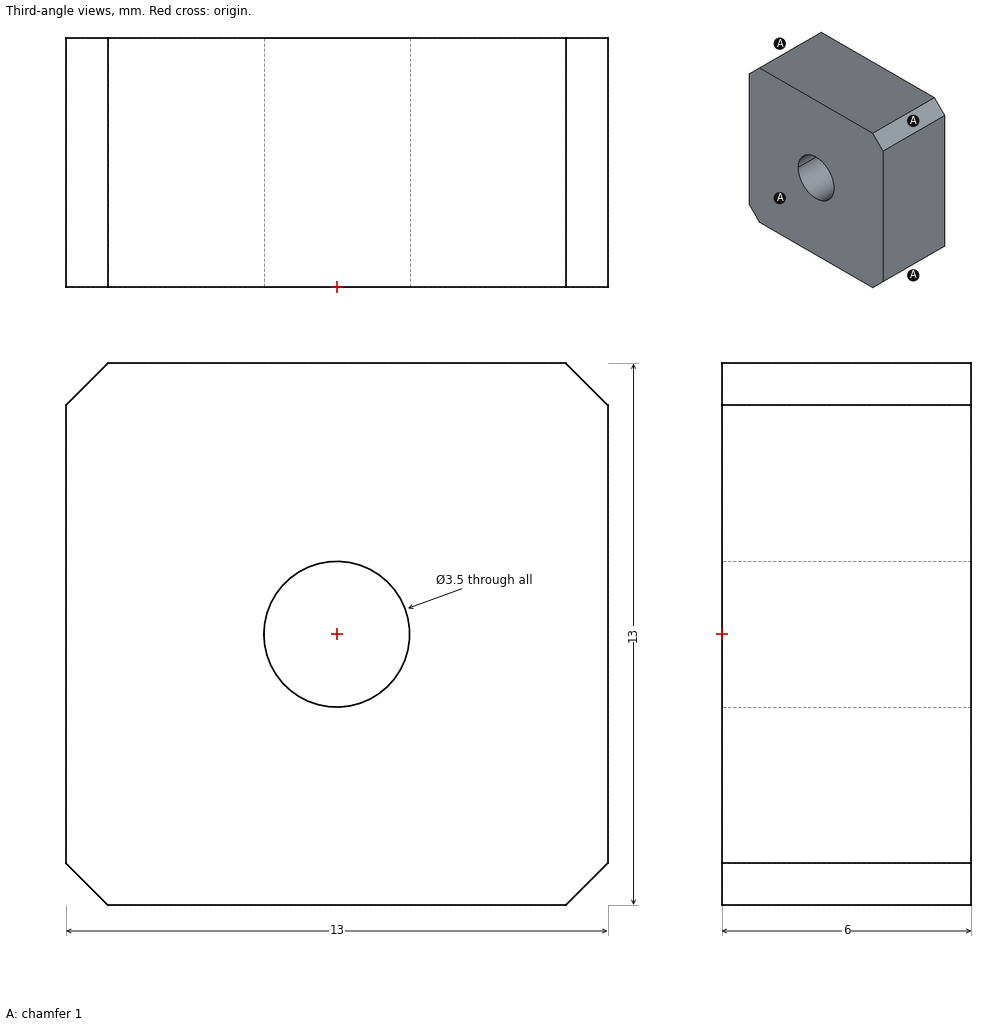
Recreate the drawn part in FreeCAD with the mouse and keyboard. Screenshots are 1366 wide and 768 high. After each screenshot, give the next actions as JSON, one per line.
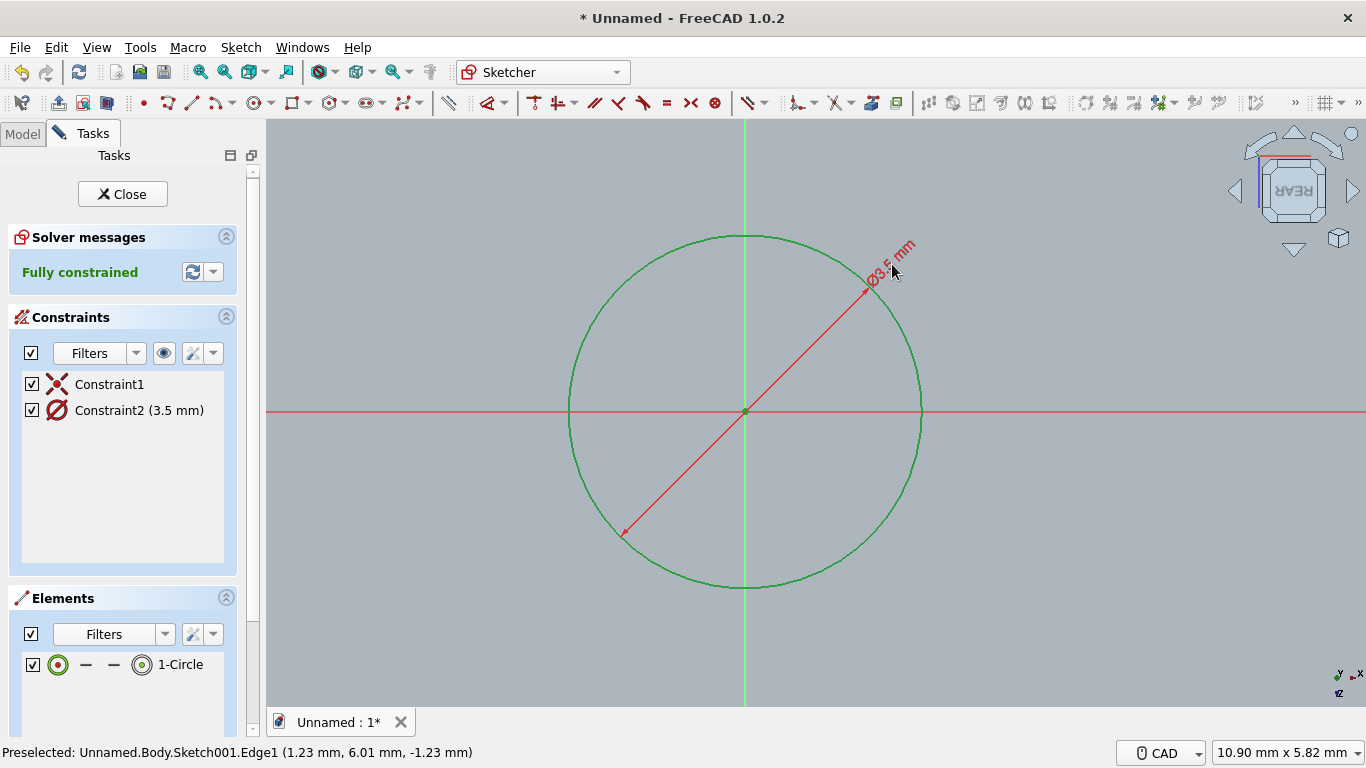
{"action": "left_click", "coordinate": [123, 194]}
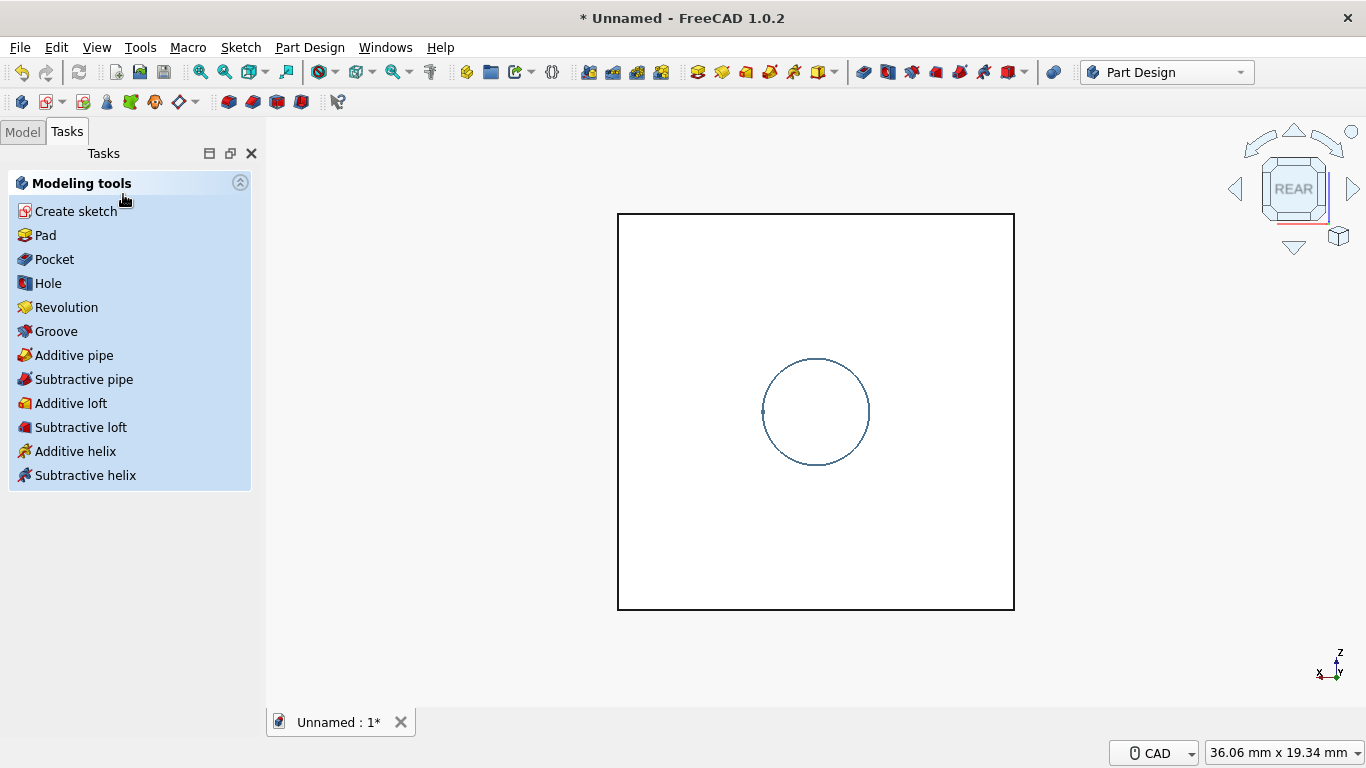
{"action": "left_click", "coordinate": [888, 72]}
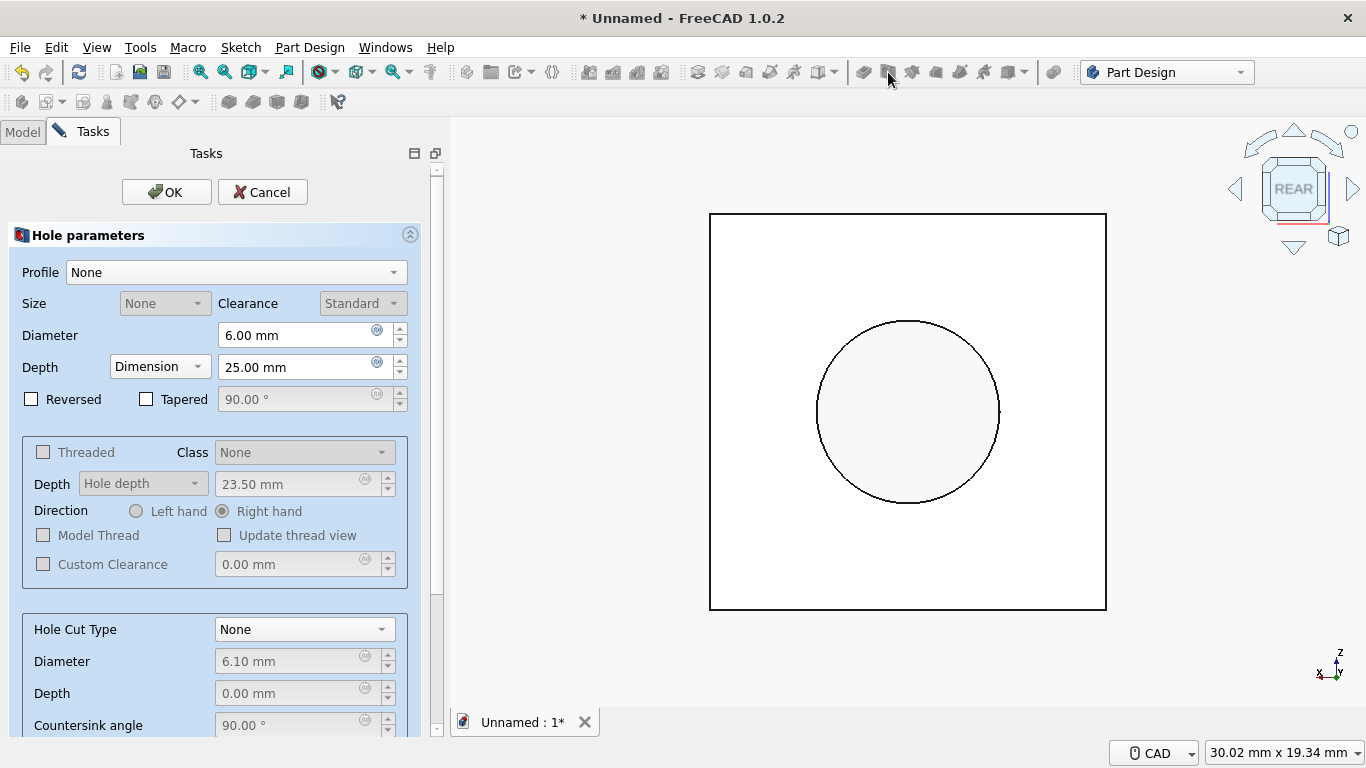
{"action": "triple_click", "coordinate": [305, 335]}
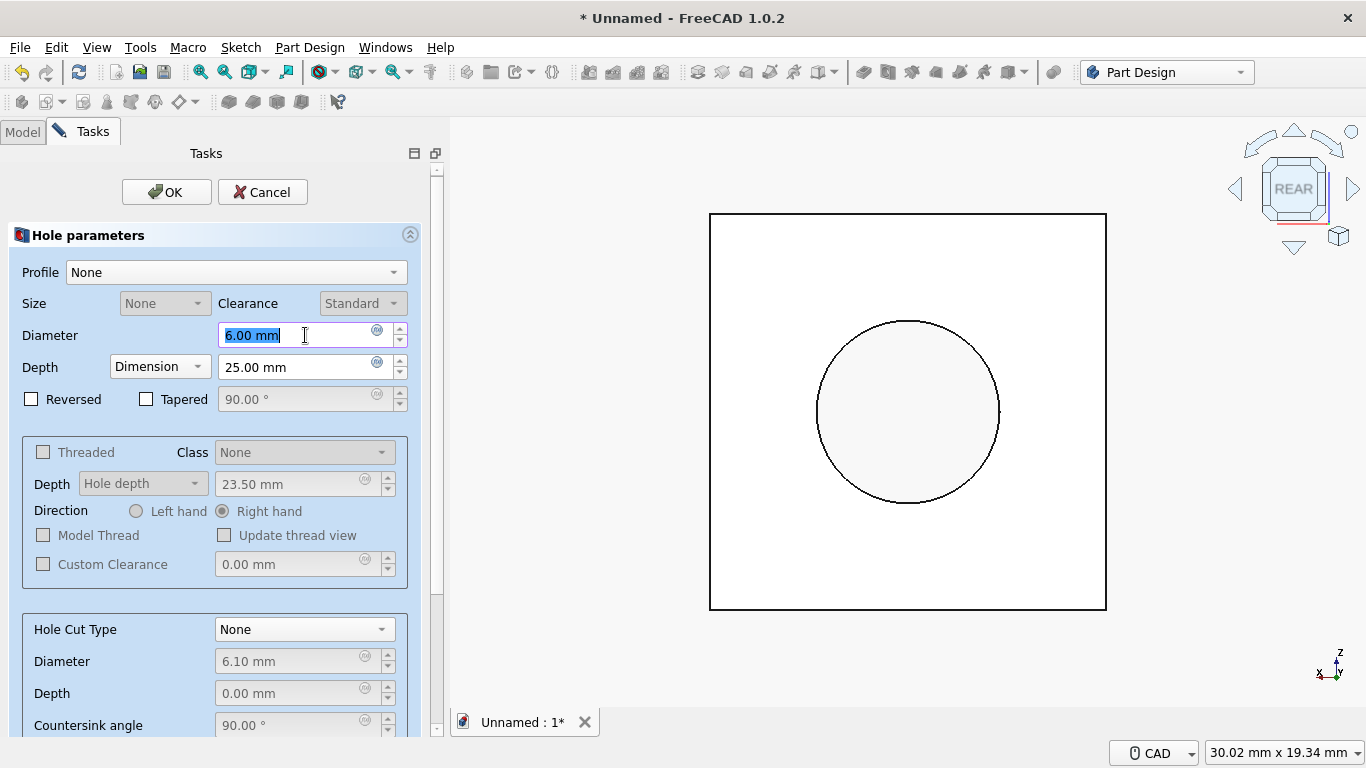
{"action": "type", "text": "3.5"}
{"action": "key", "text": "Tab"}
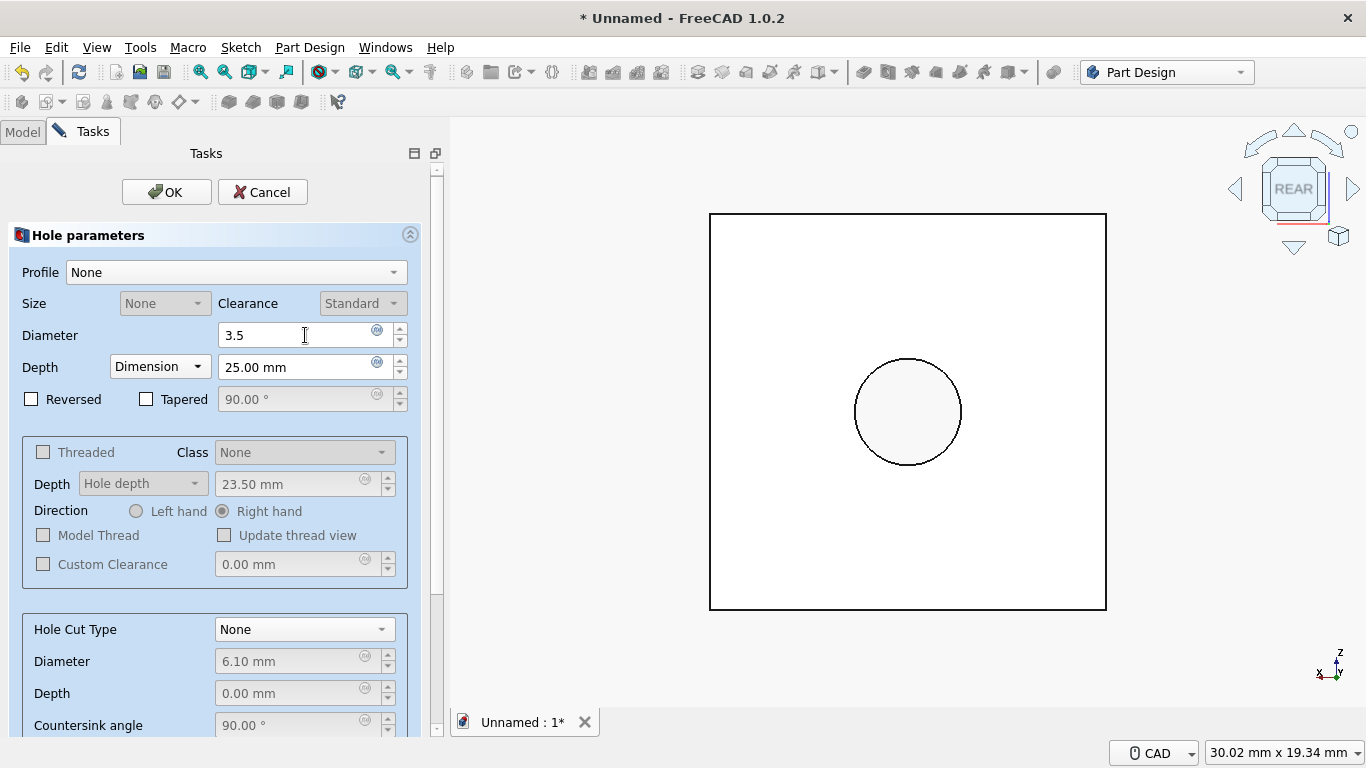
{"action": "left_click", "coordinate": [161, 366]}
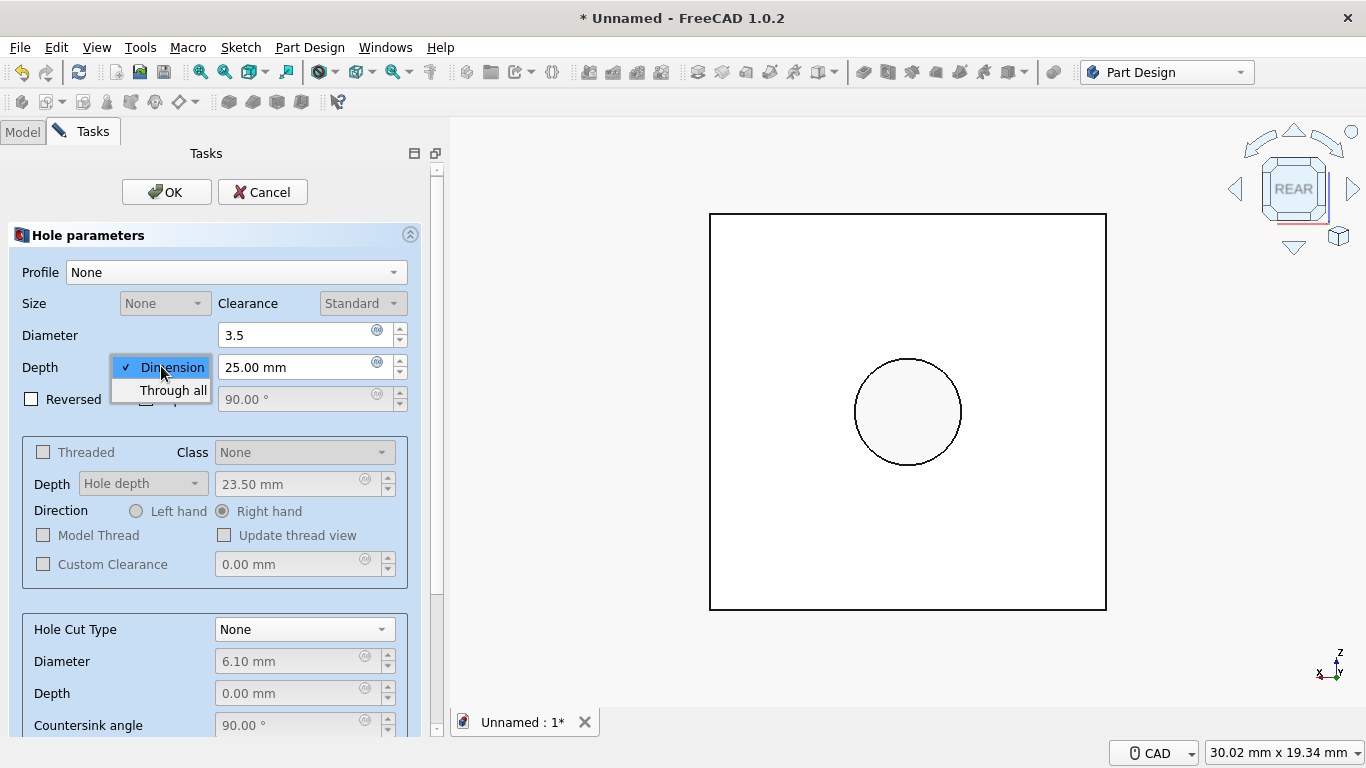
{"action": "left_click", "coordinate": [160, 390]}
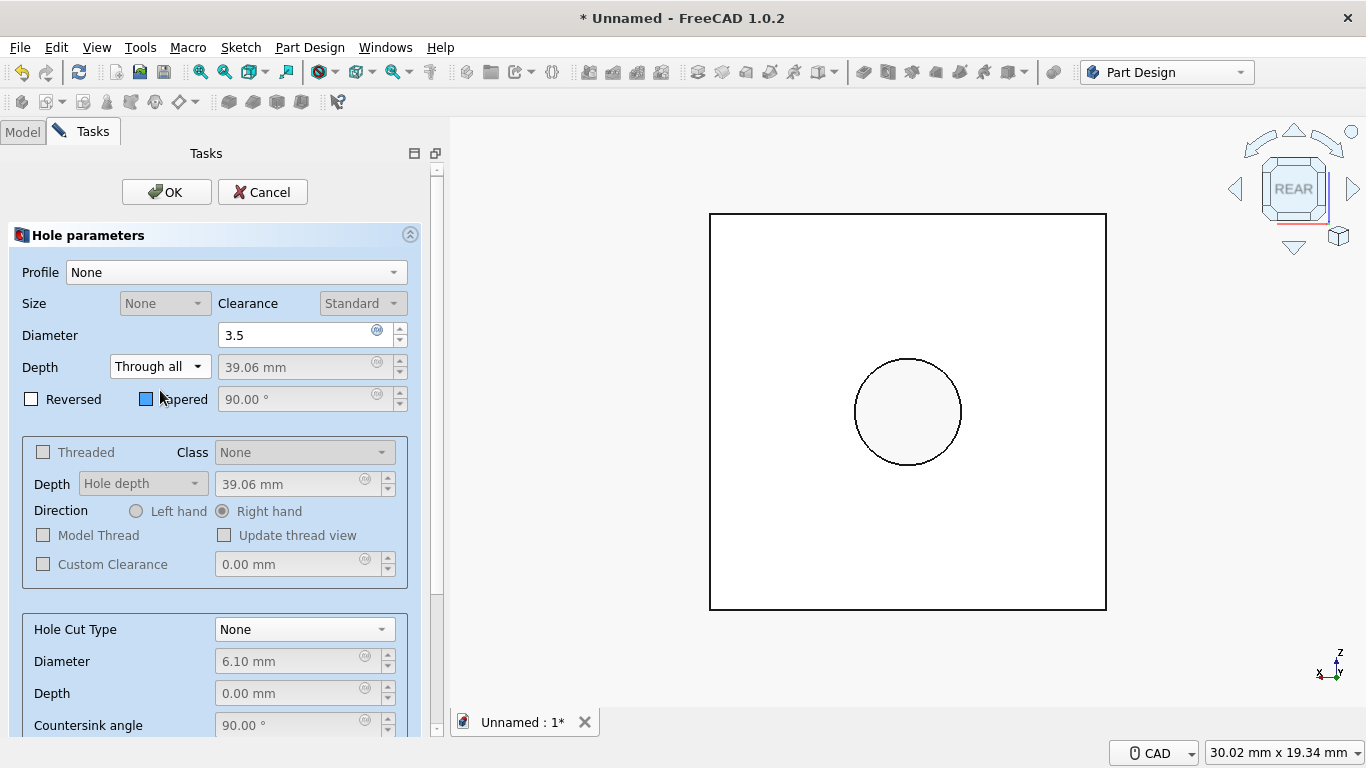
{"action": "left_click", "coordinate": [167, 192]}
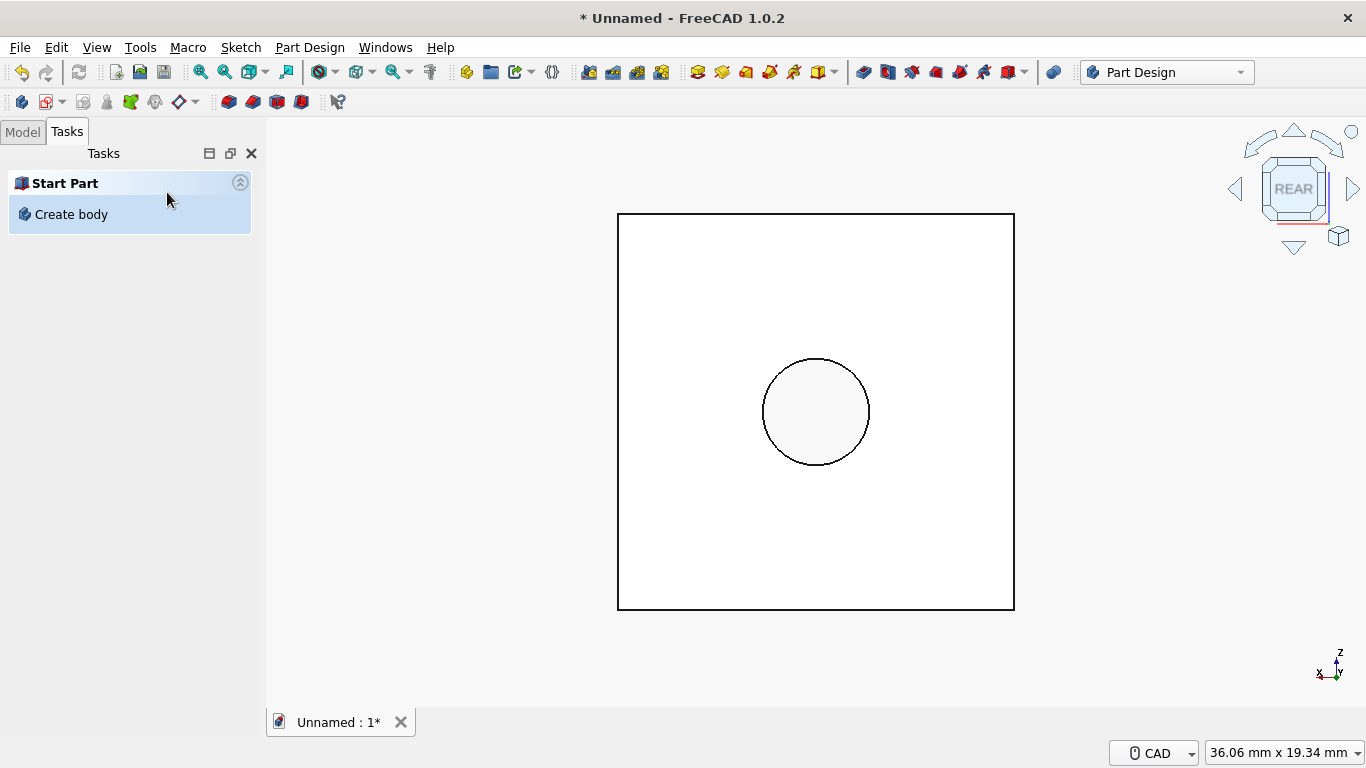
{"action": "key", "text": "0"}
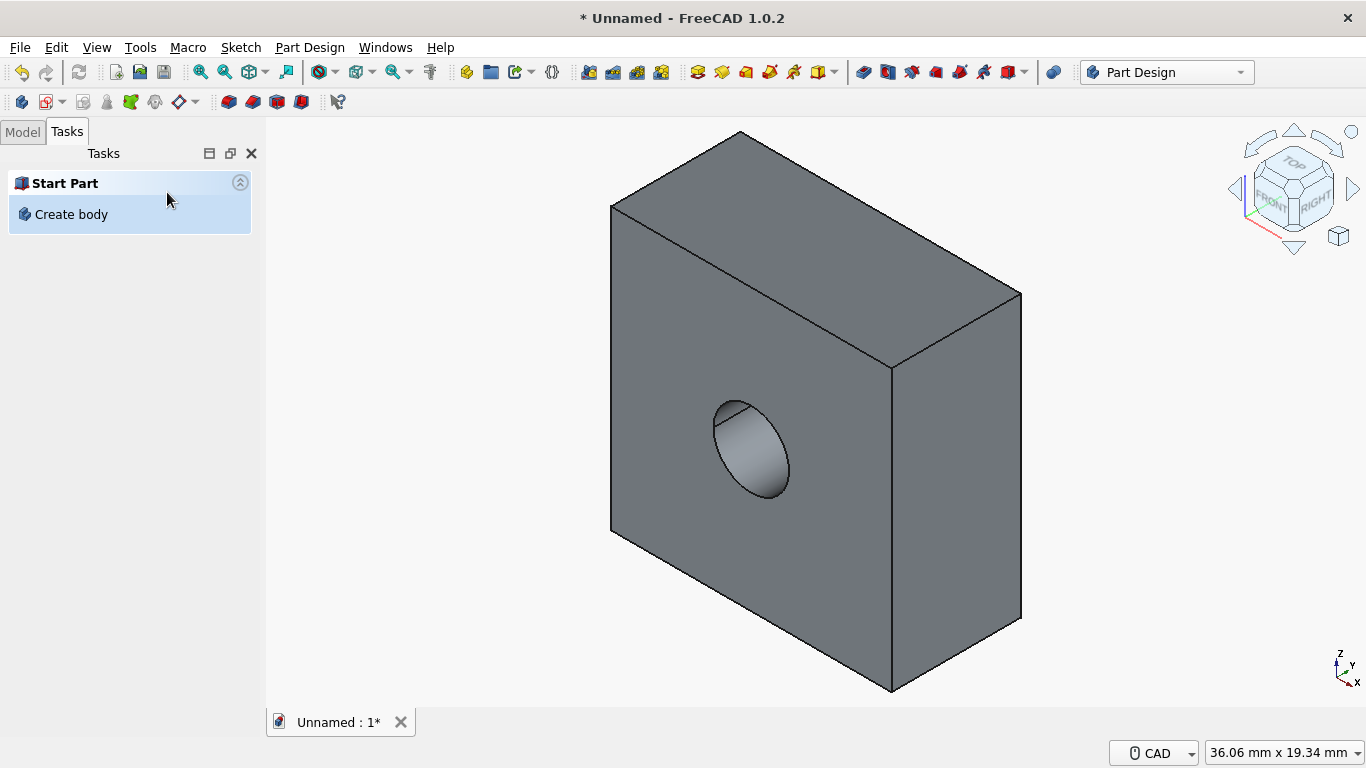
{"action": "left_click", "coordinate": [956, 330]}